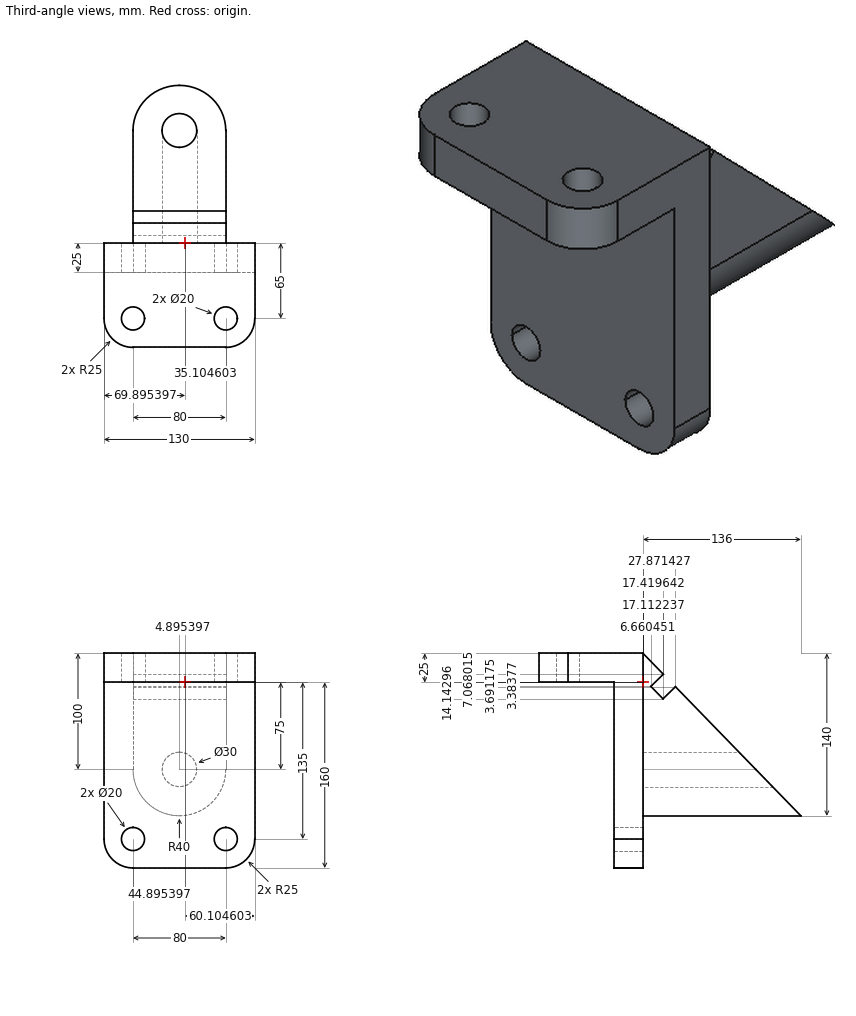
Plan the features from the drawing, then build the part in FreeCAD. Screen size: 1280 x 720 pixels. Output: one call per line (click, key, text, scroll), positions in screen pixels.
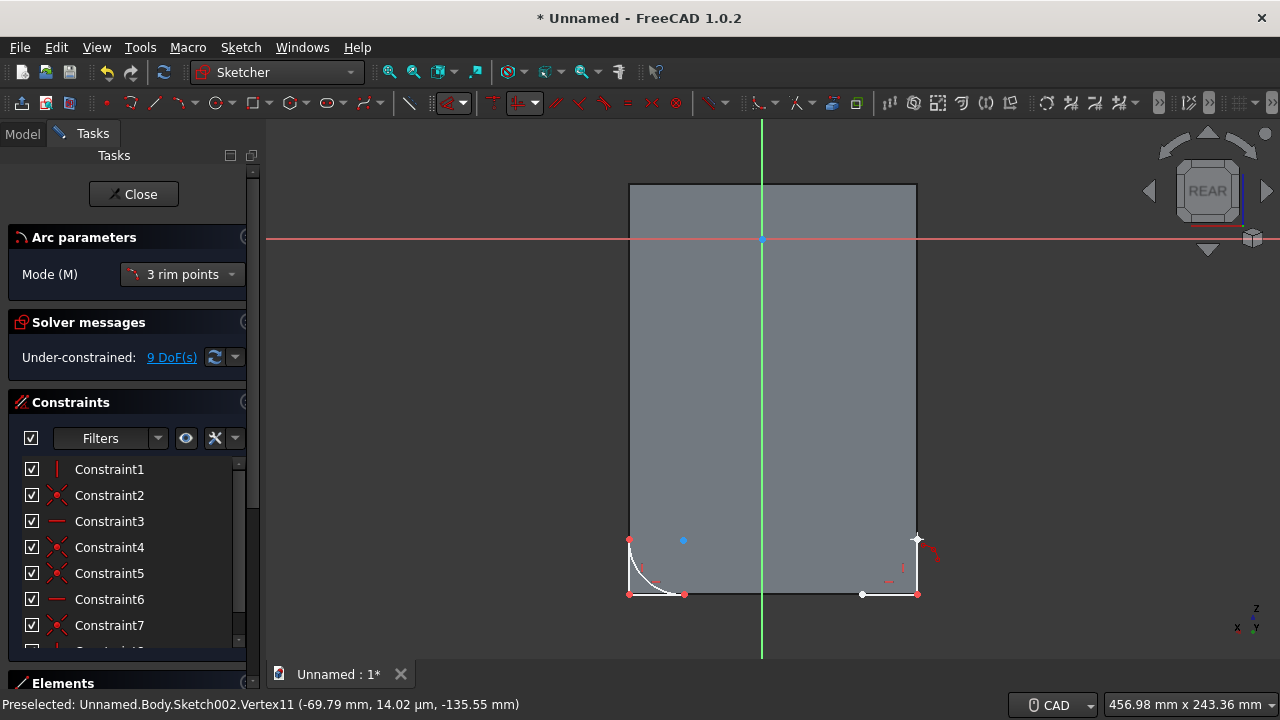
click(917, 540)
click(862, 595)
click(901, 578)
key(Escape)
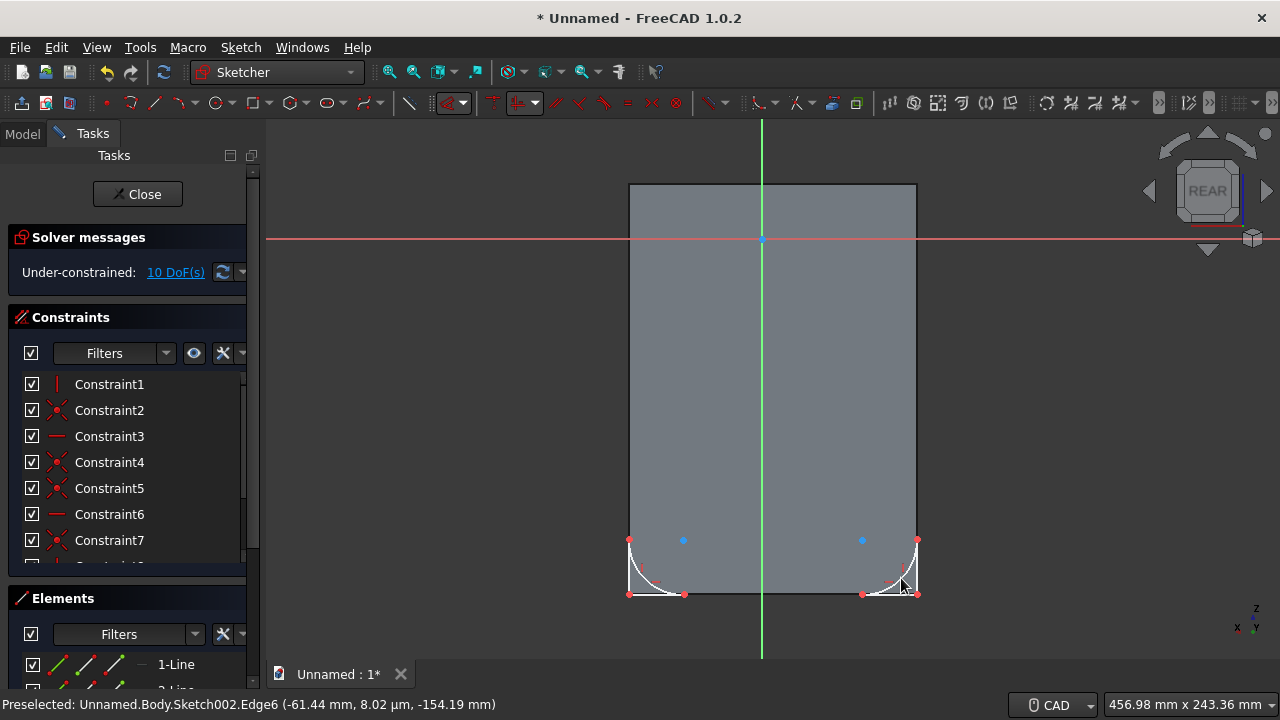
click(629, 578)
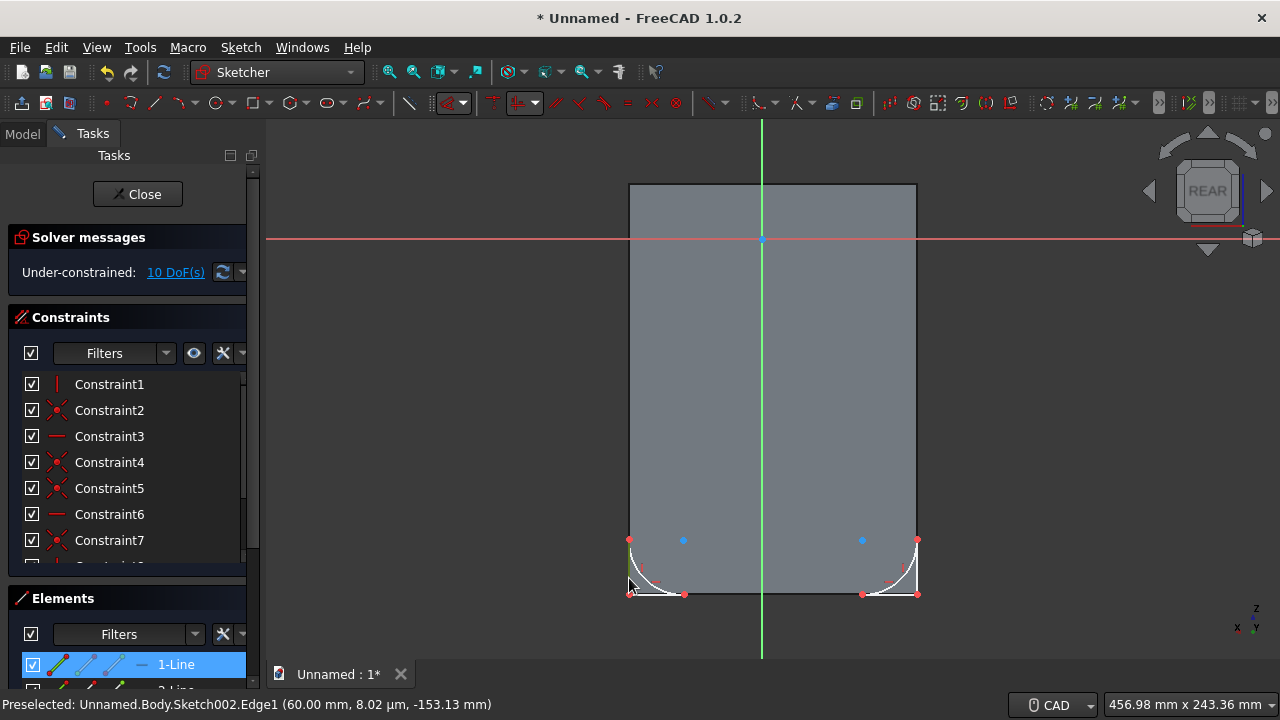
click(645, 579)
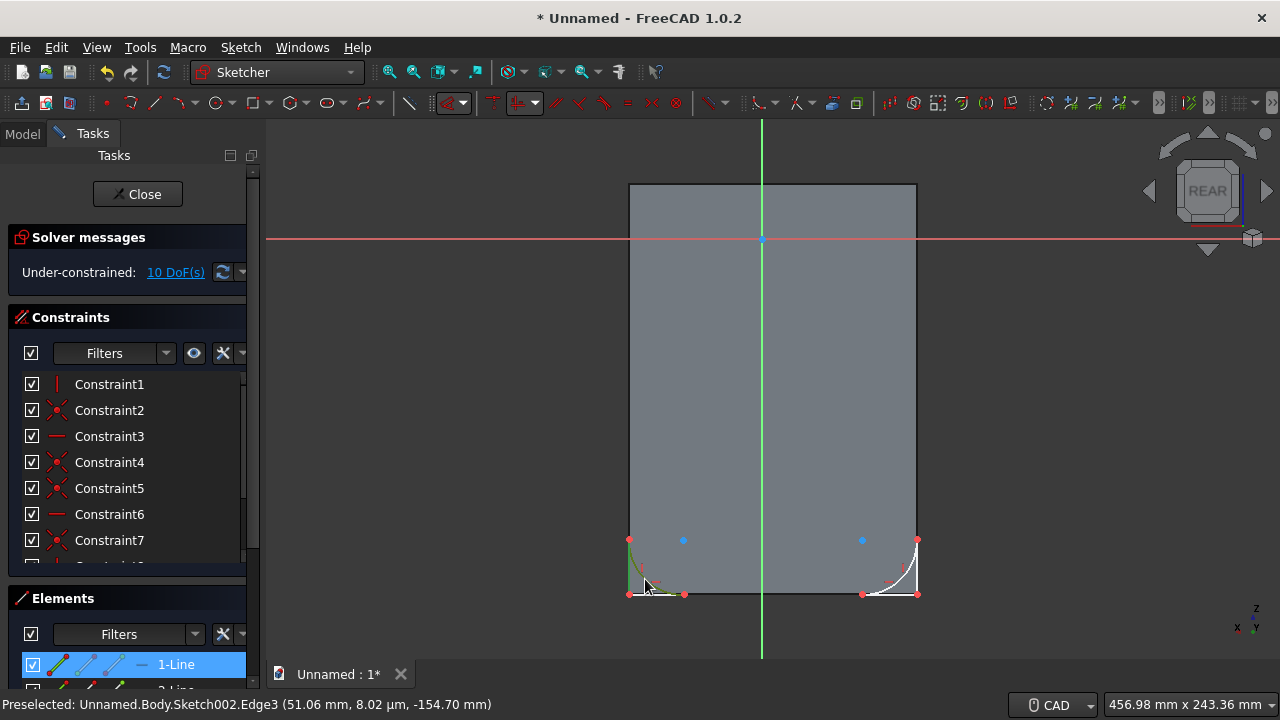
click(604, 104)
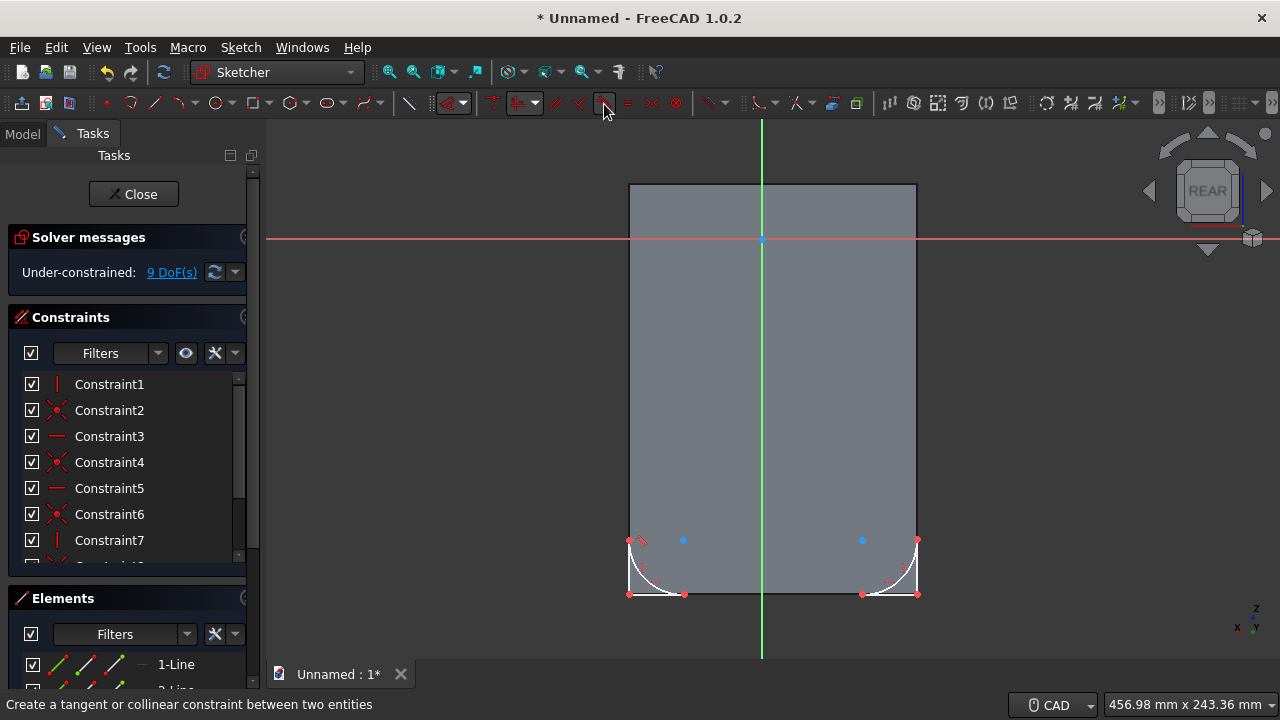
click(646, 595)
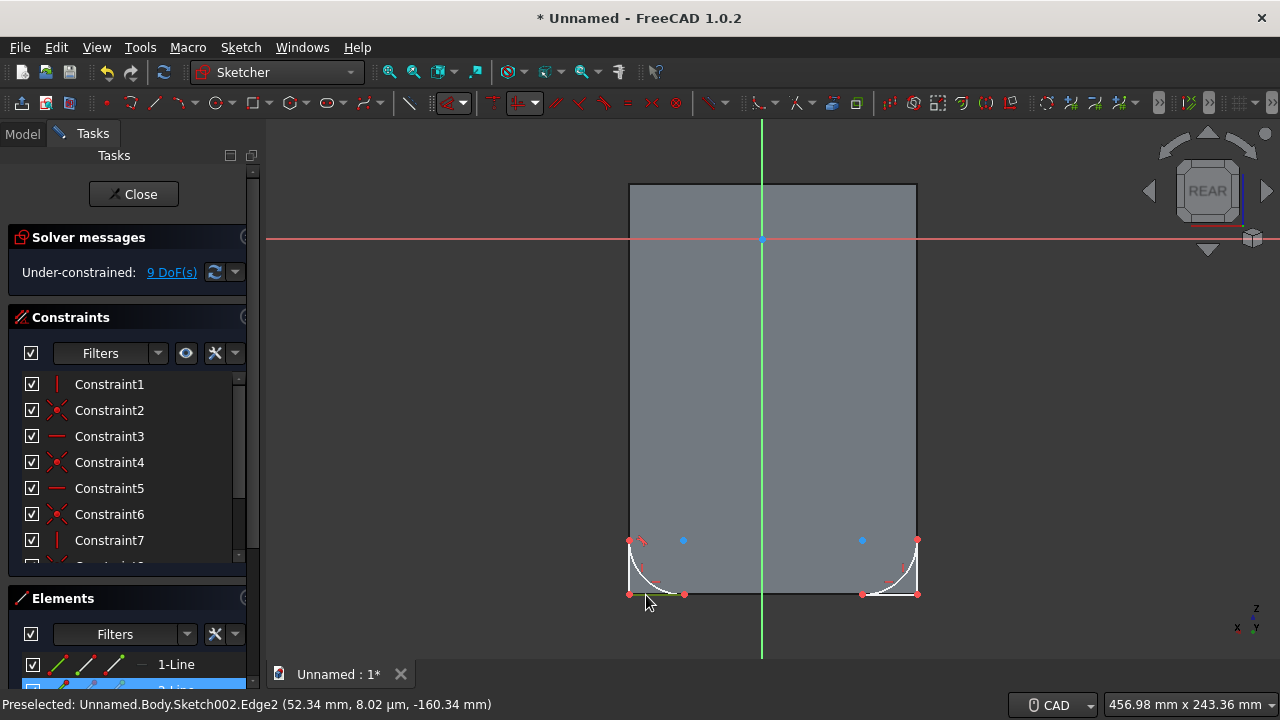
click(645, 579)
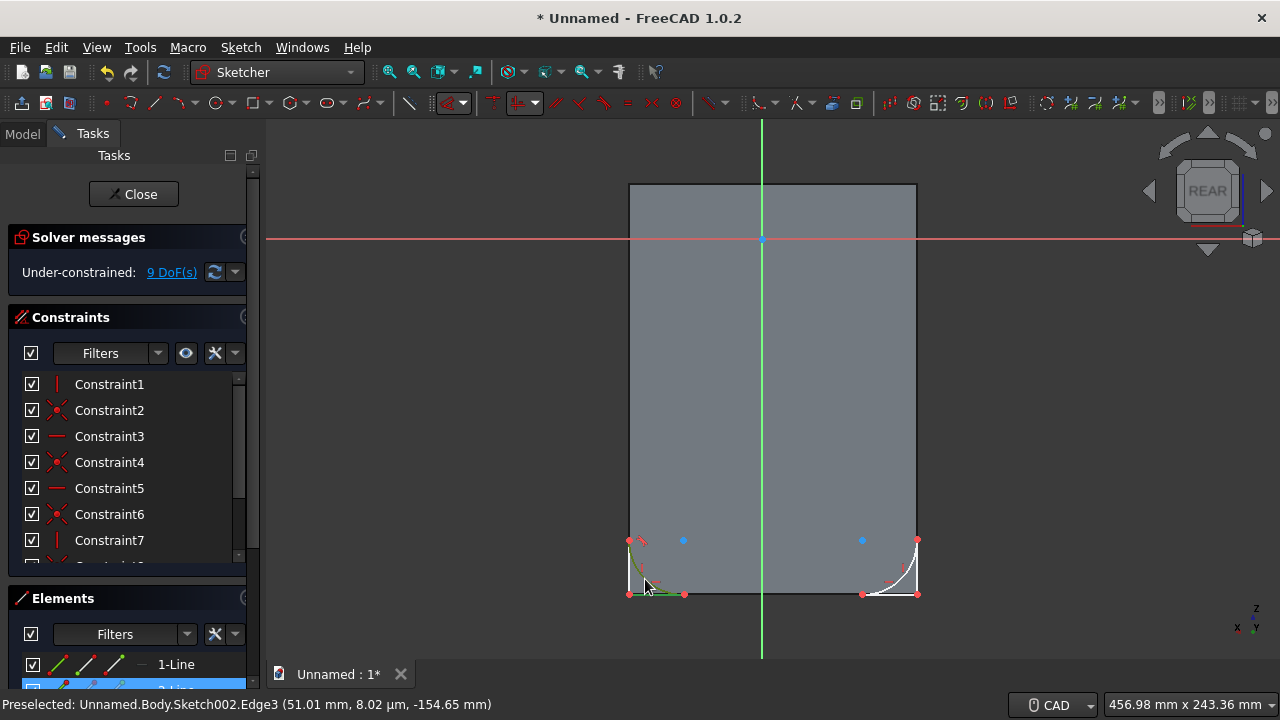
key(t)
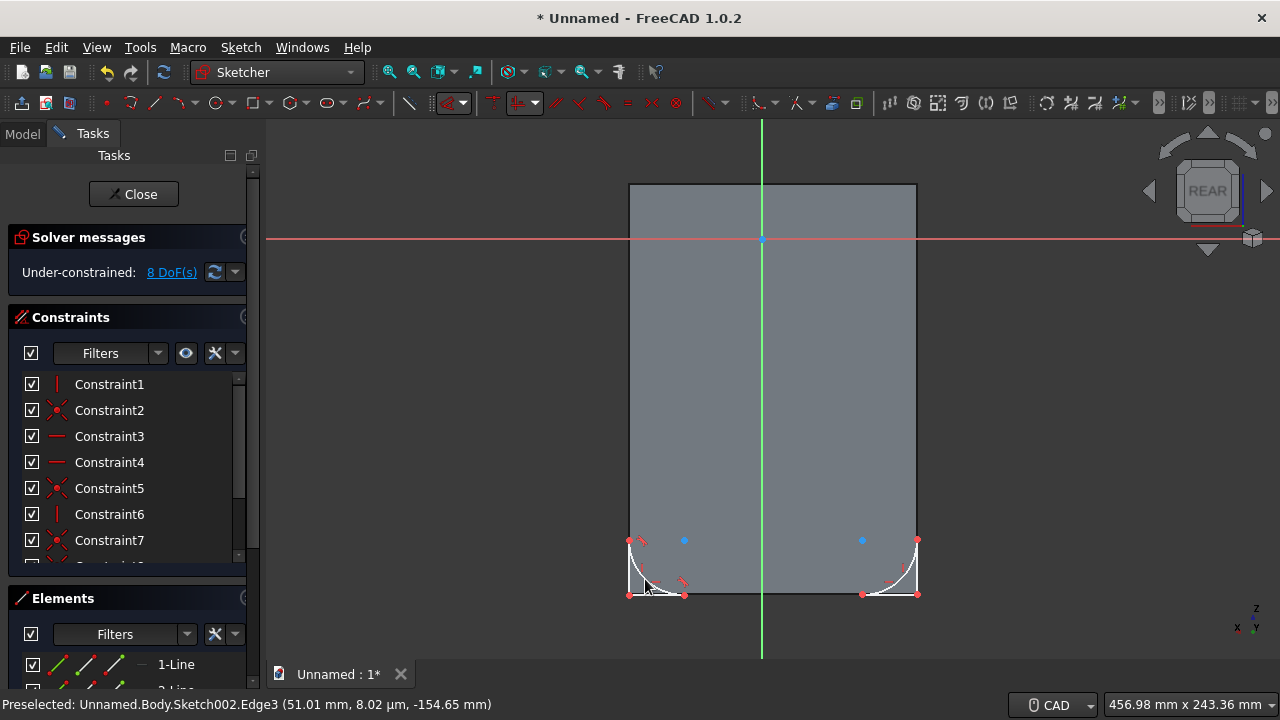
click(900, 595)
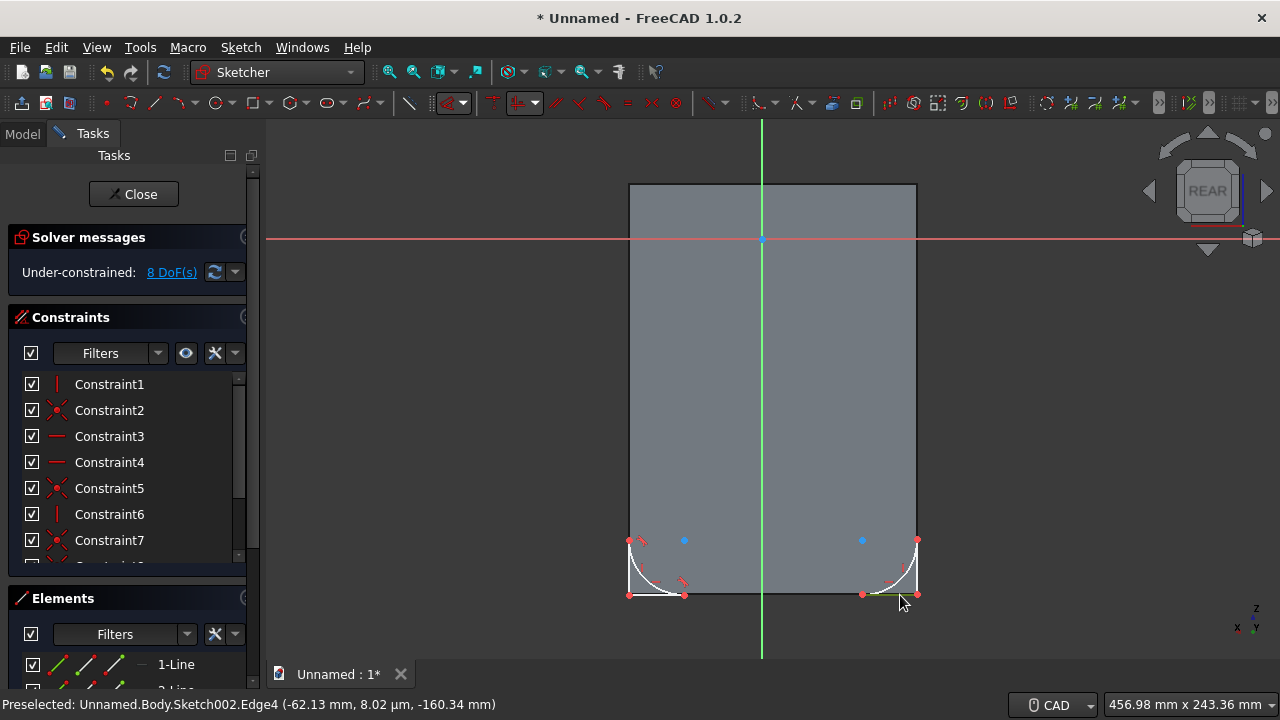
click(901, 579)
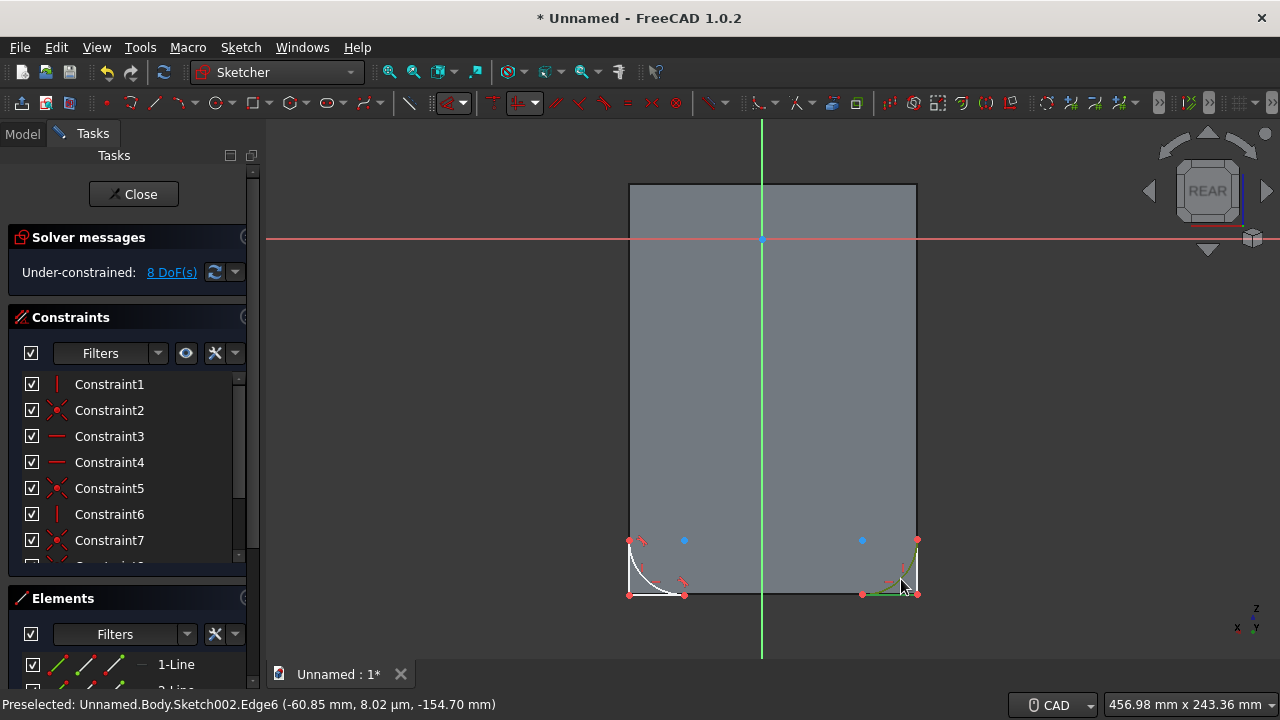
click(604, 104)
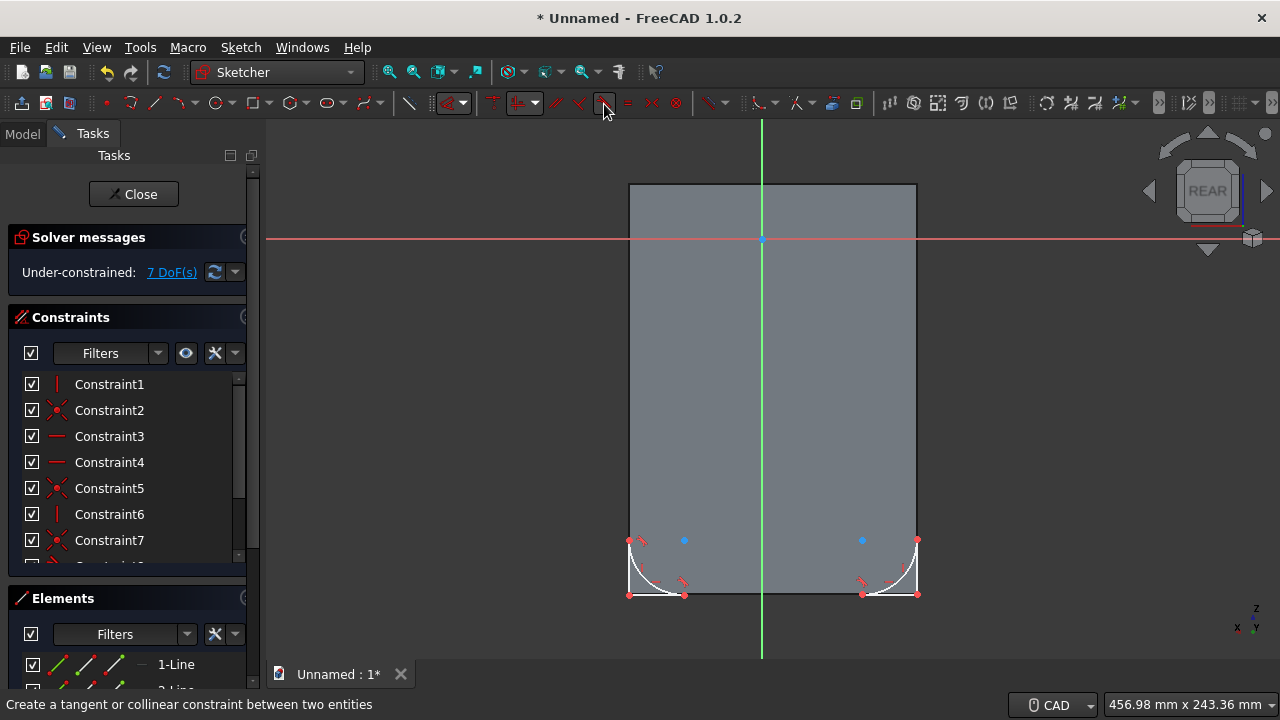
click(917, 578)